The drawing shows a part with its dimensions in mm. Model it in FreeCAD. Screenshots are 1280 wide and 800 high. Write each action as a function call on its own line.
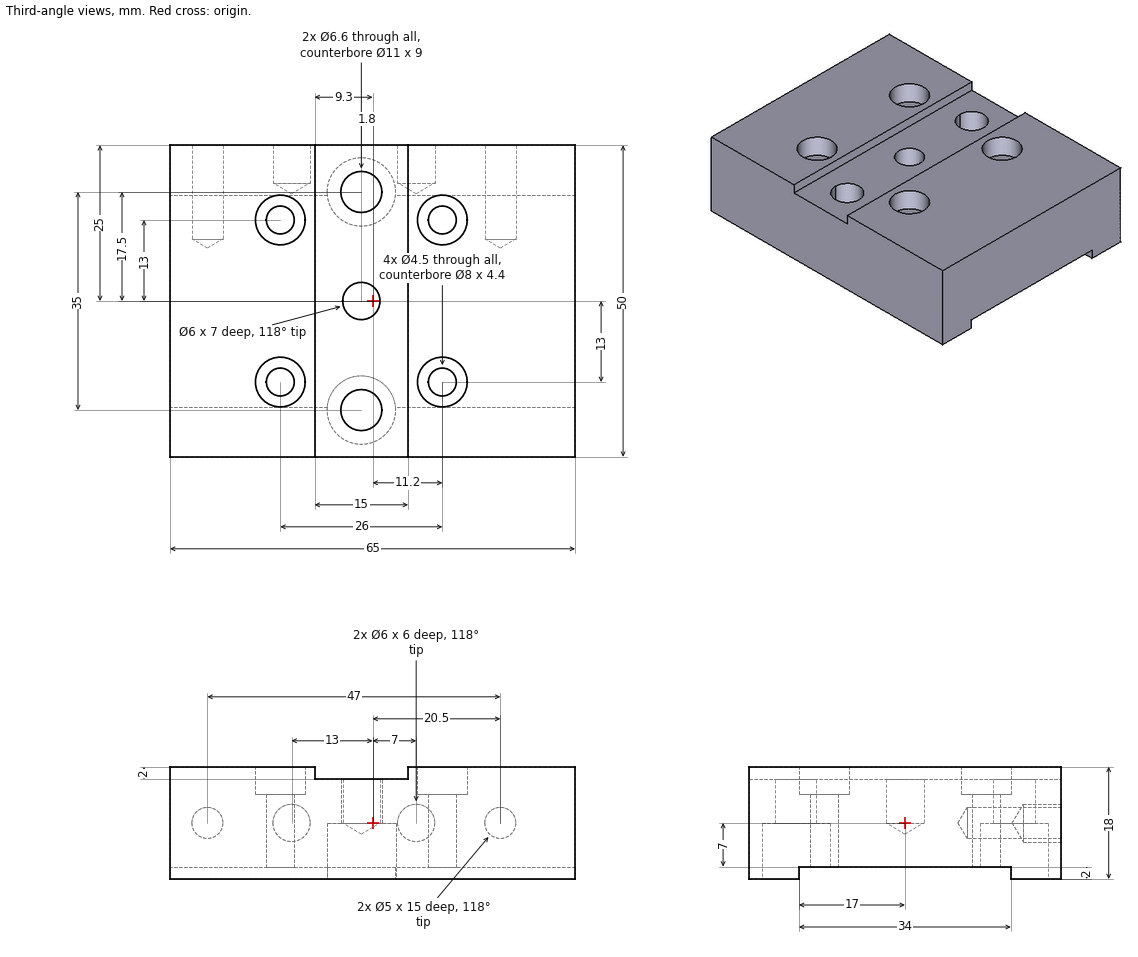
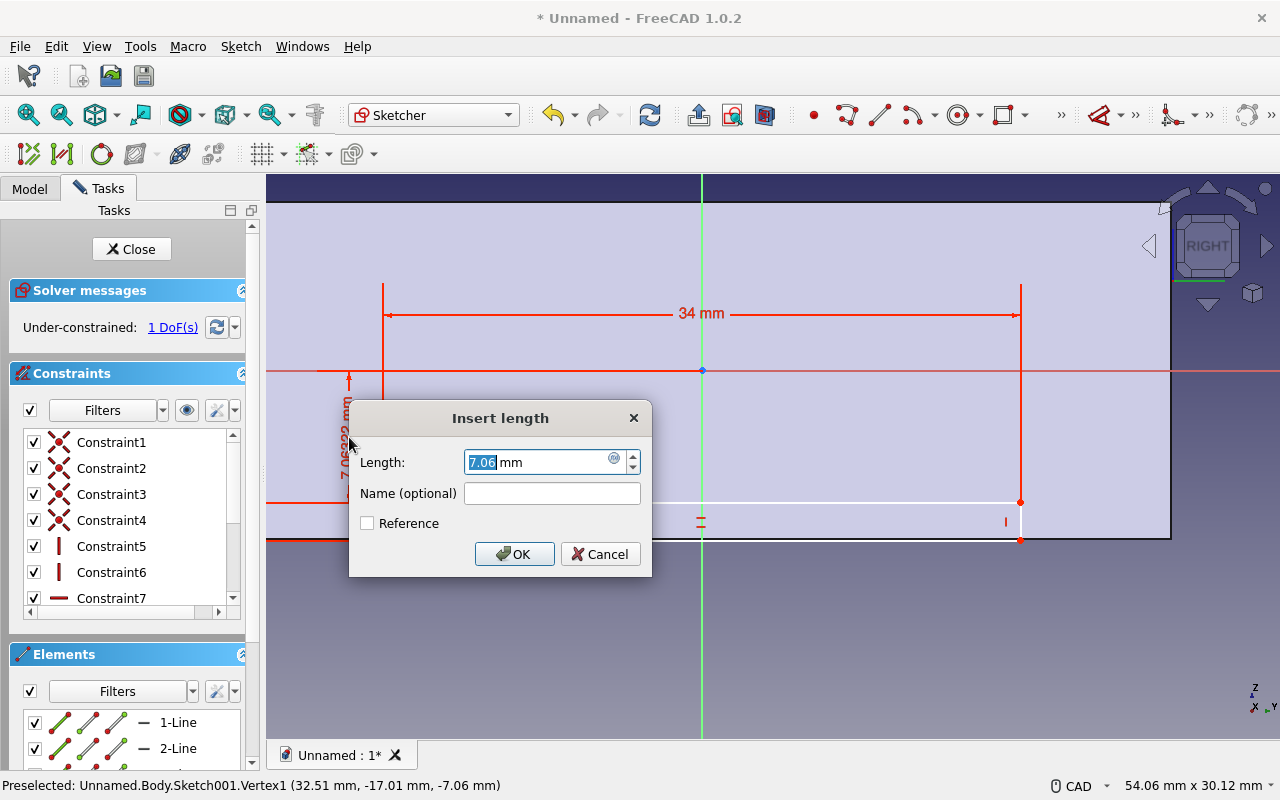
text(7)
key(Return)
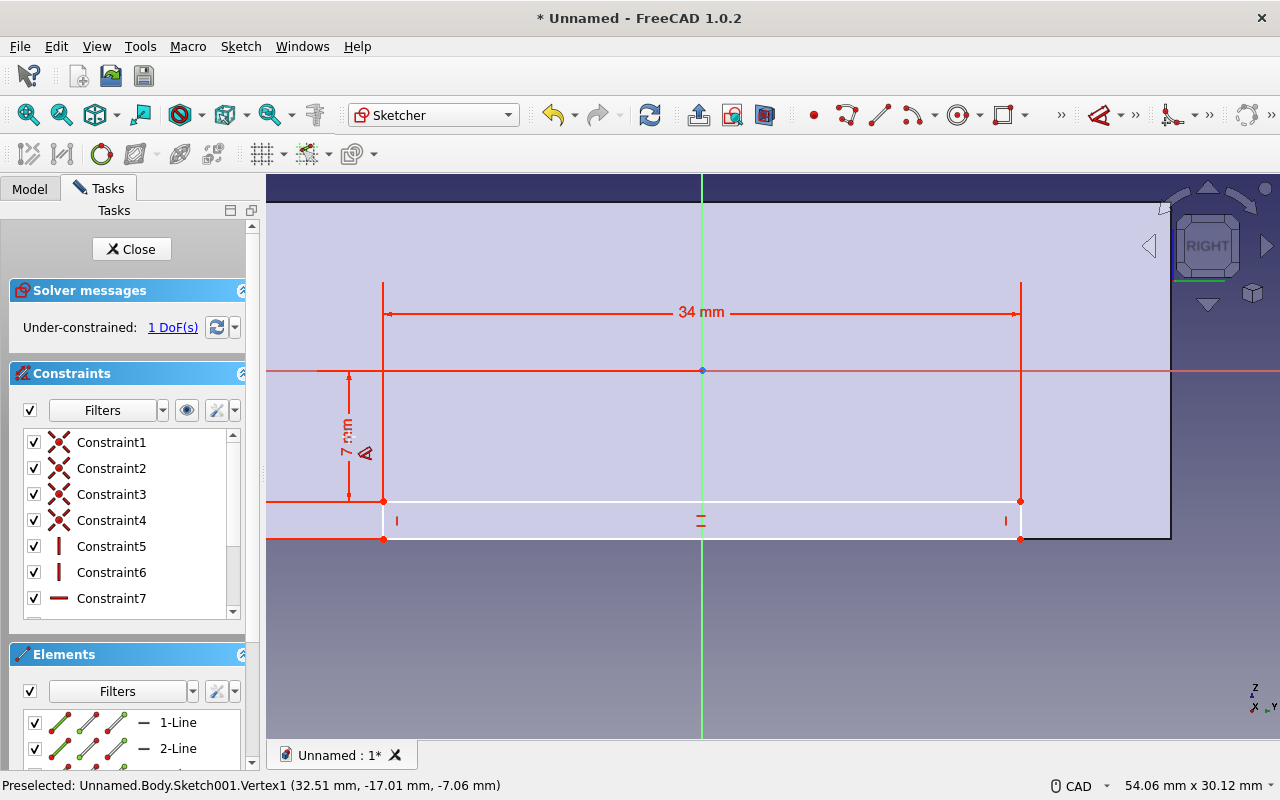
click(383, 502)
click(543, 337)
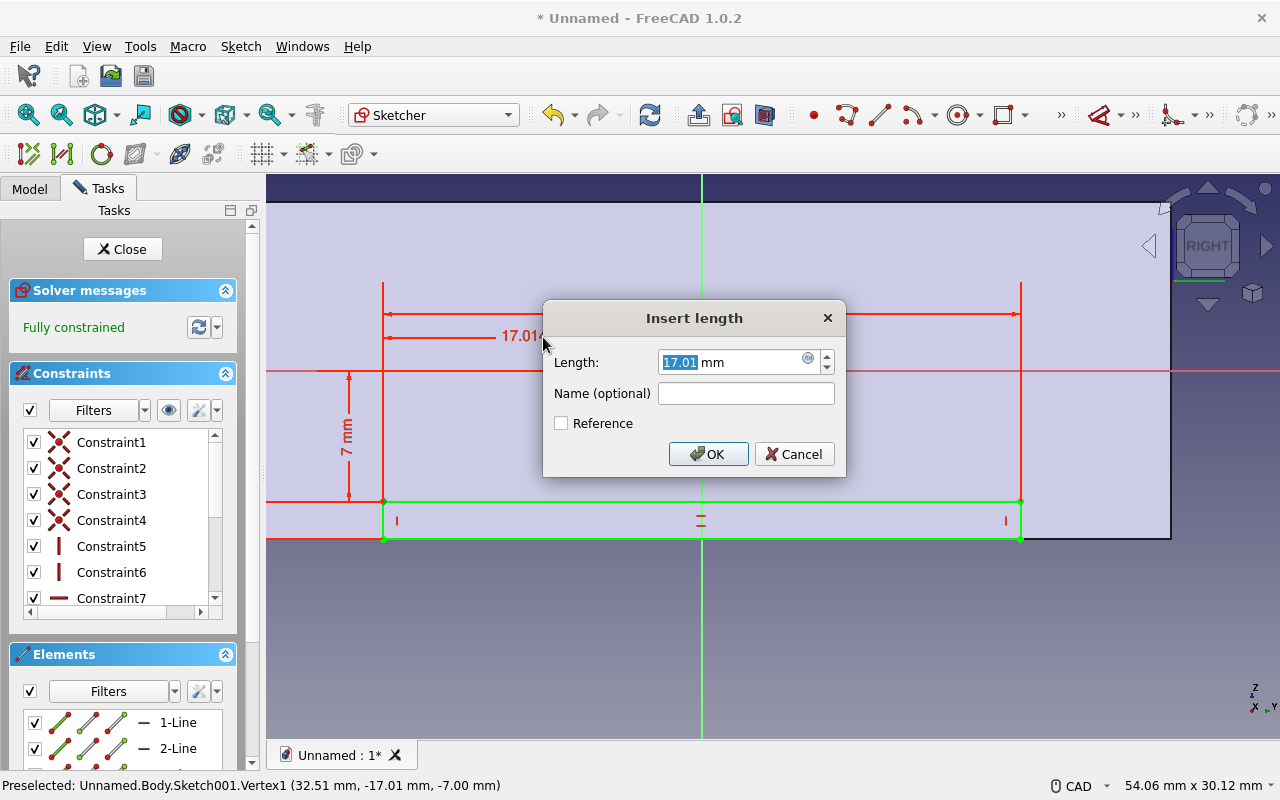
text(17)
key(Return)
key(Escape)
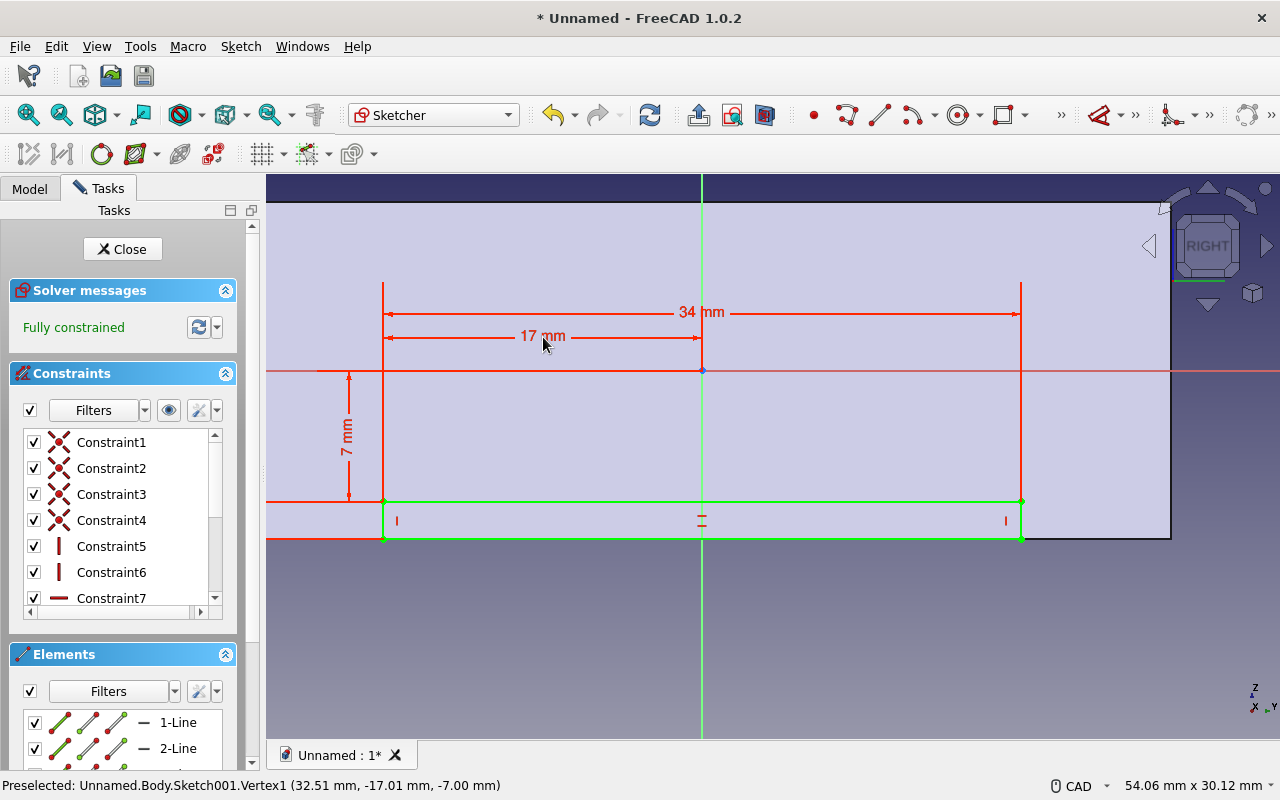
click(123, 249)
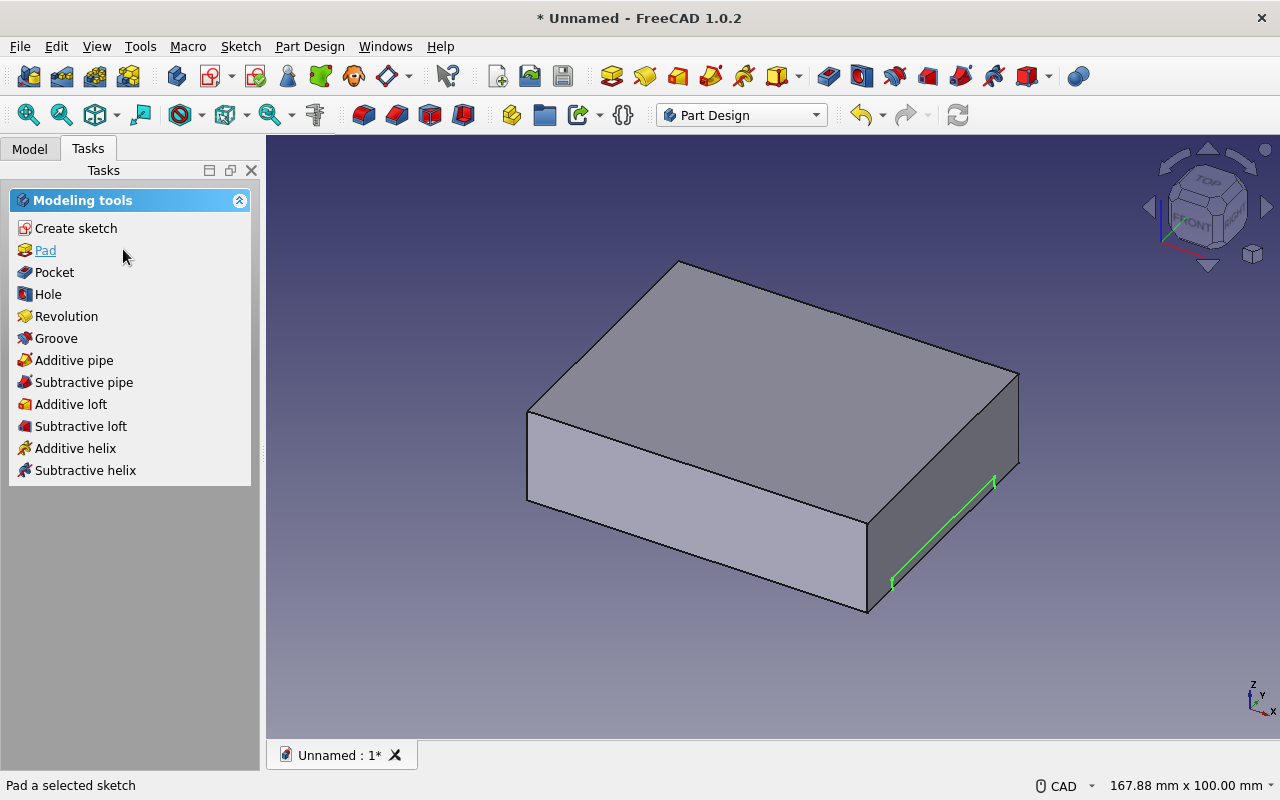
click(829, 76)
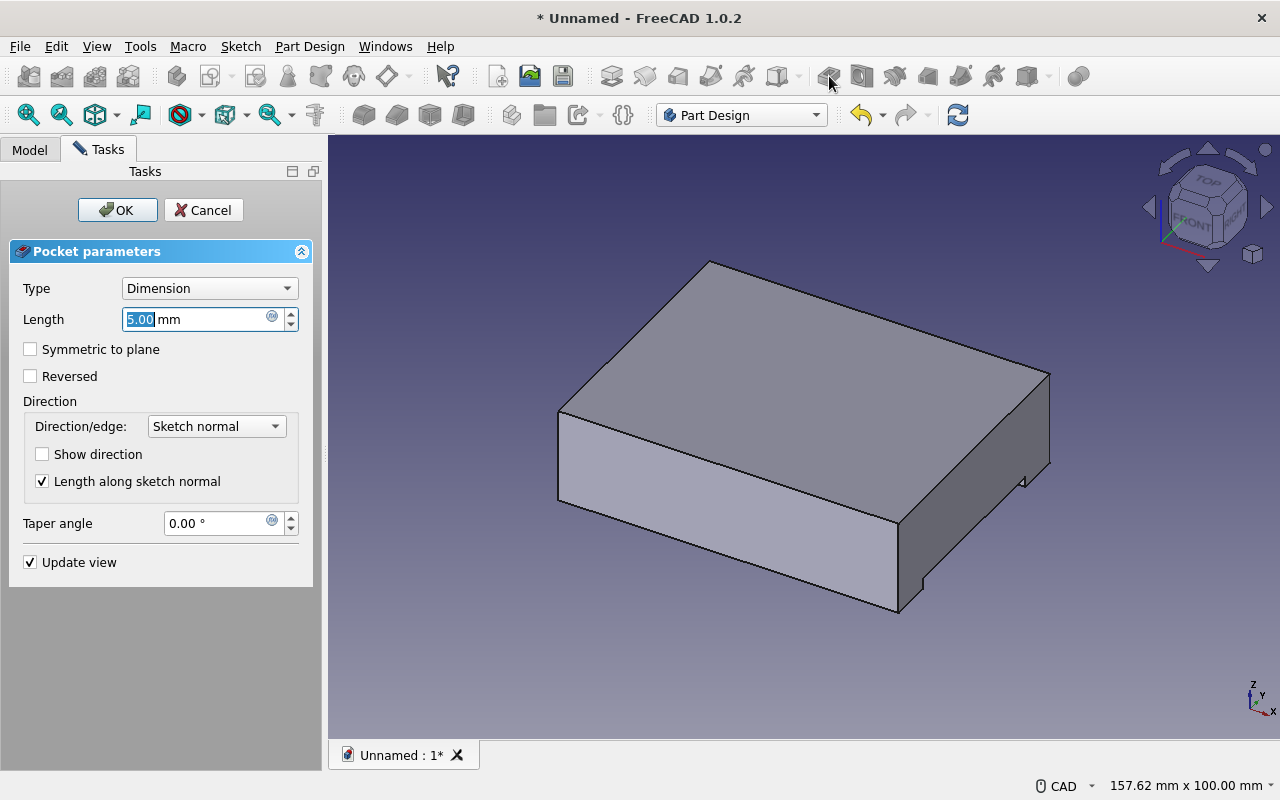
click(210, 288)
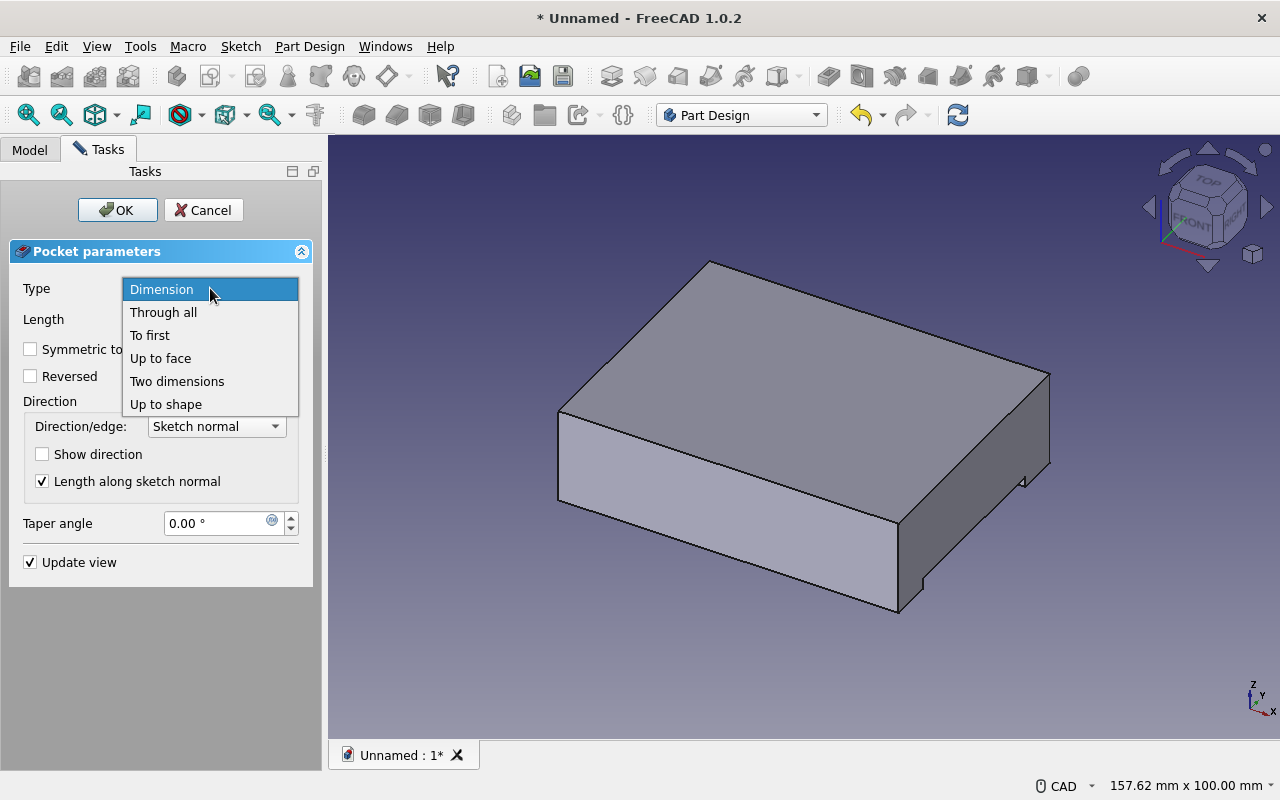
click(208, 312)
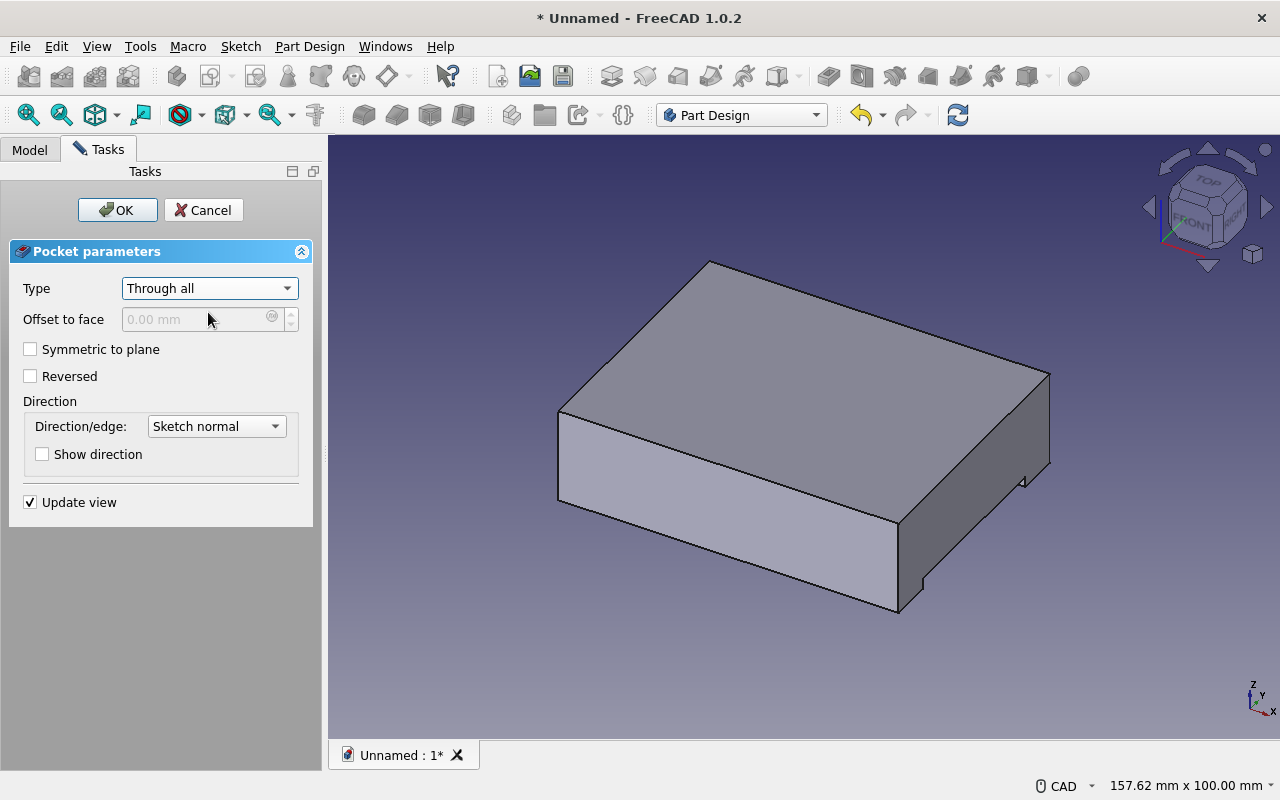
click(118, 210)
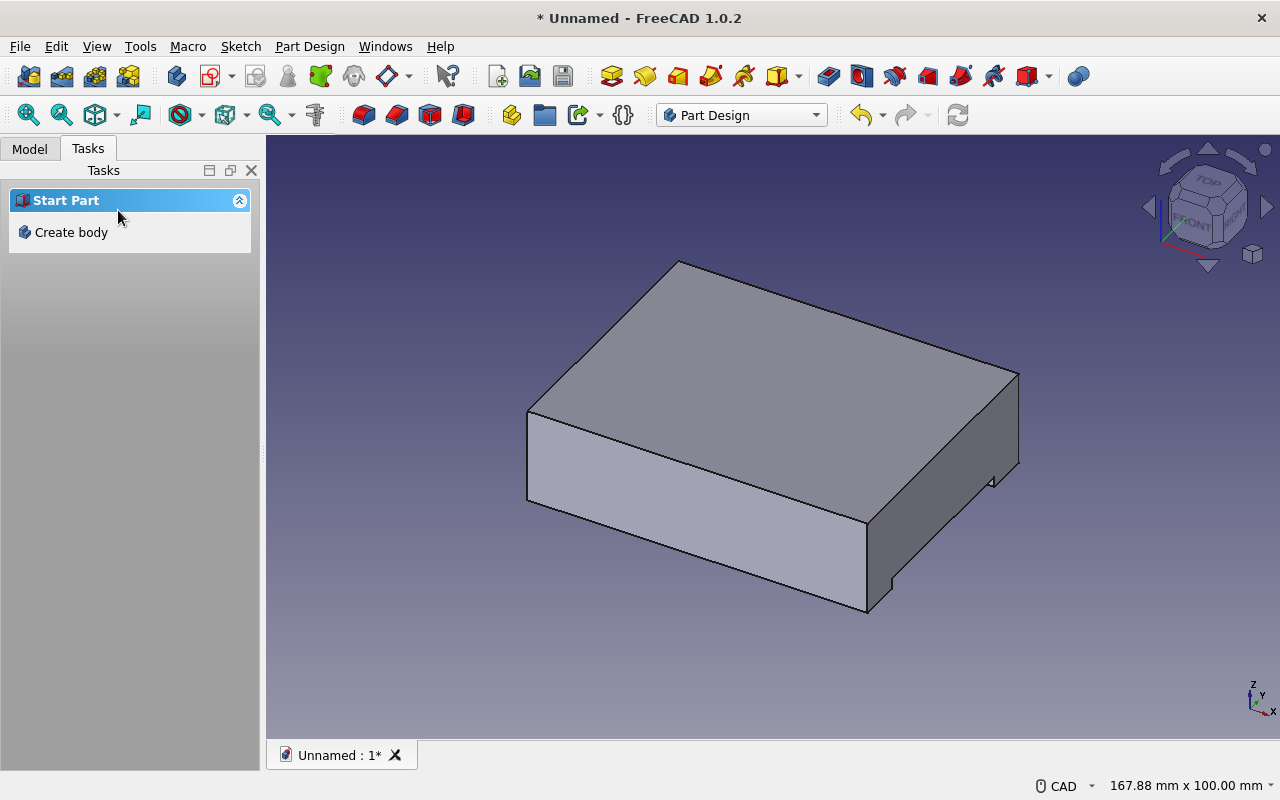
click(773, 391)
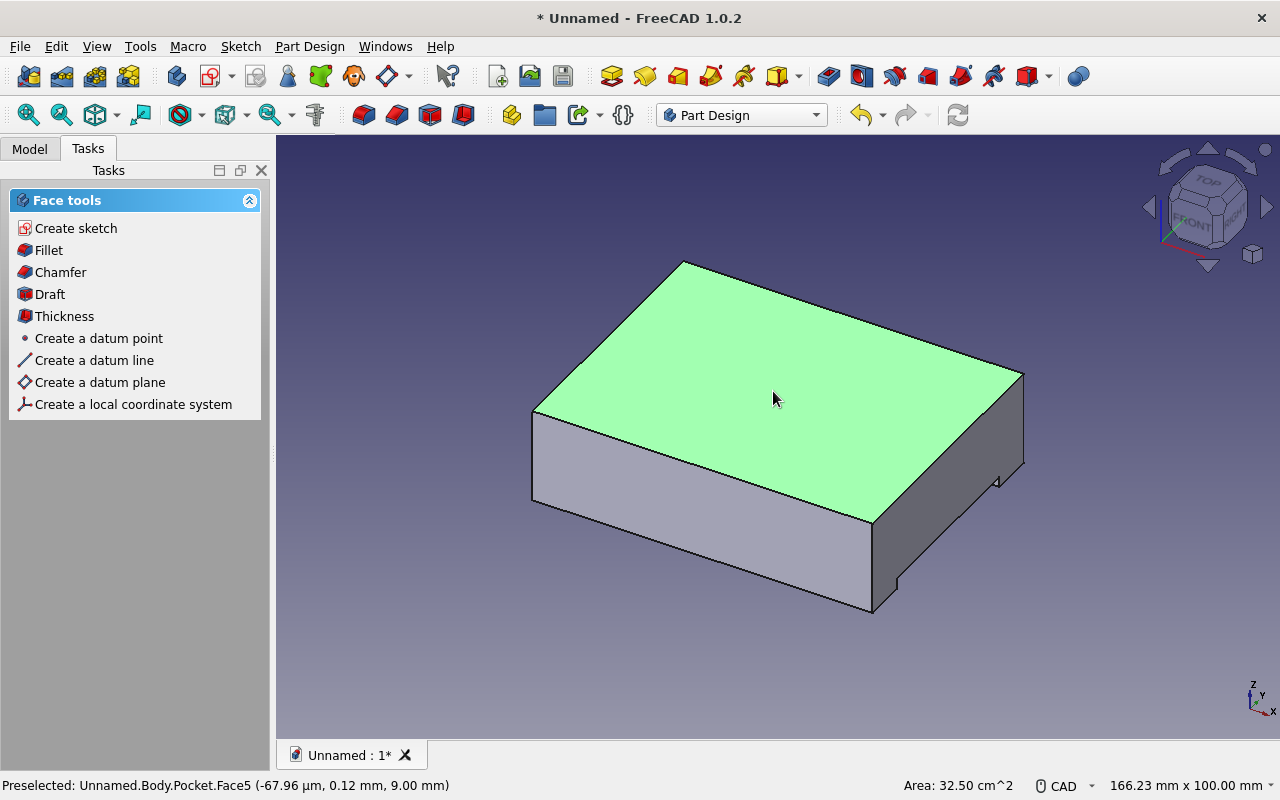
click(210, 76)